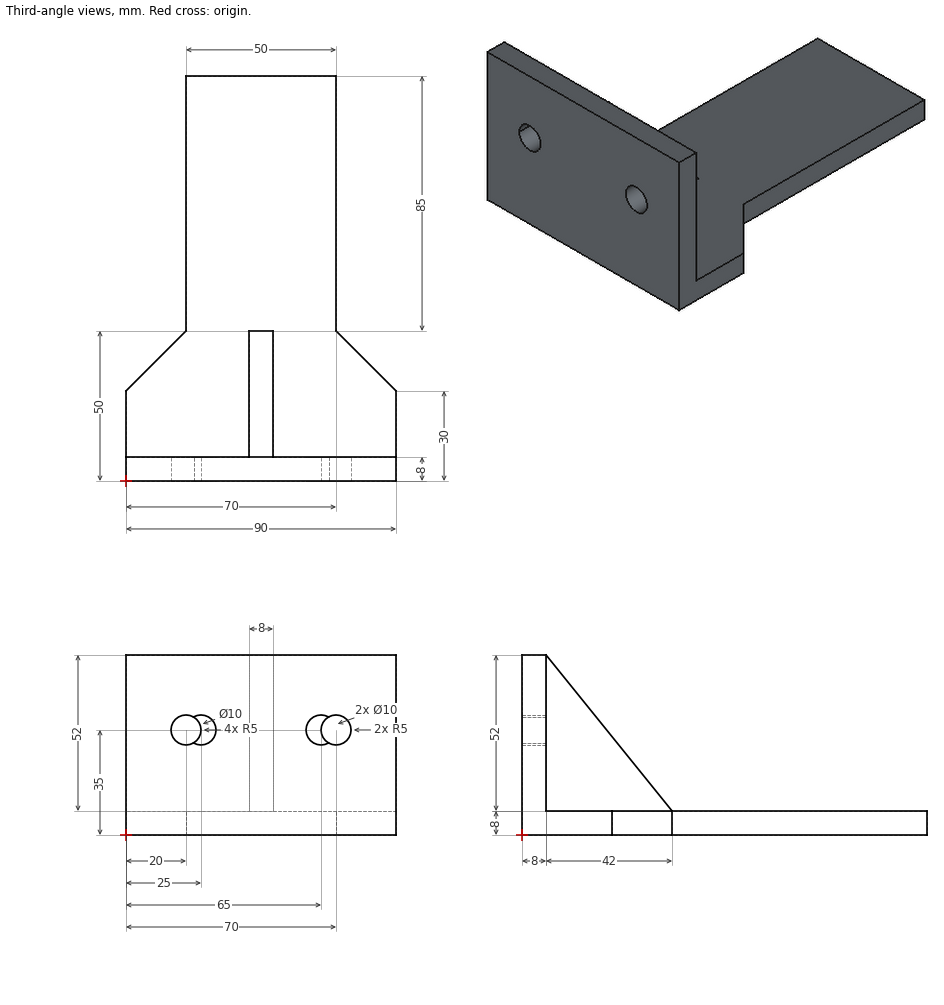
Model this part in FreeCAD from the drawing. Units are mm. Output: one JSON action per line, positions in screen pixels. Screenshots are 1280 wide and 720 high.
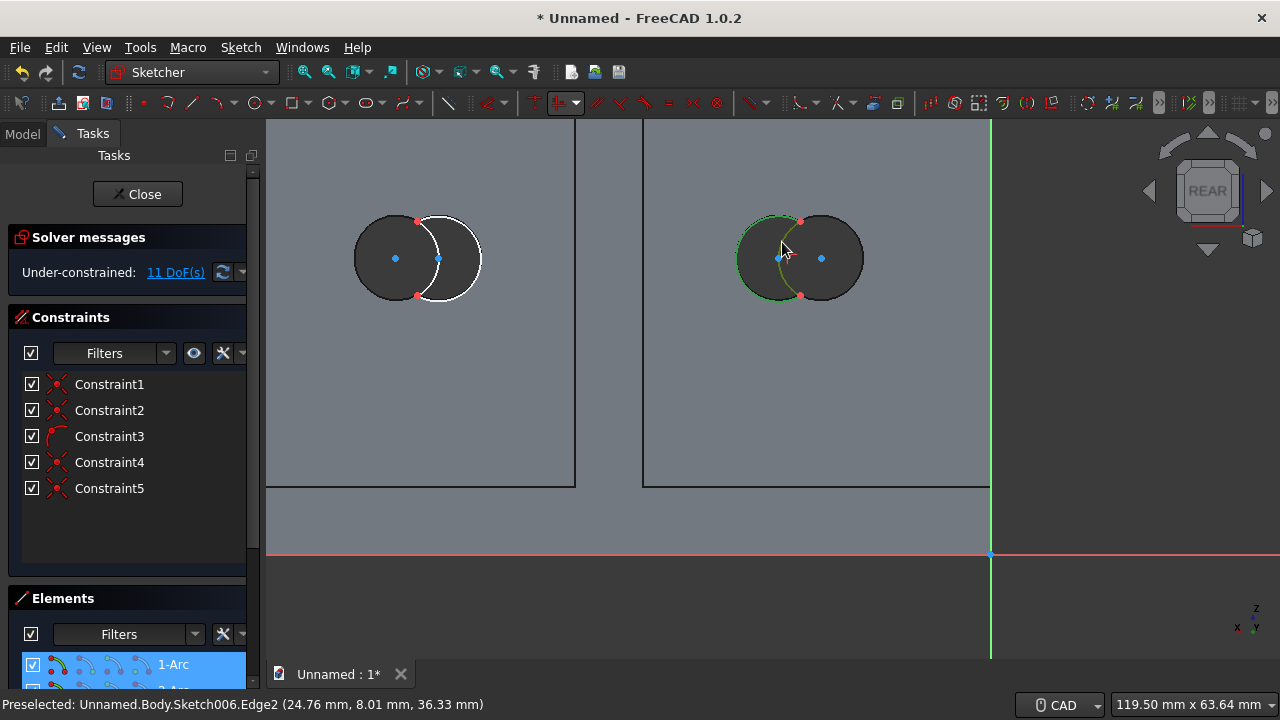
{"action": "left_click", "coordinate": [435, 276]}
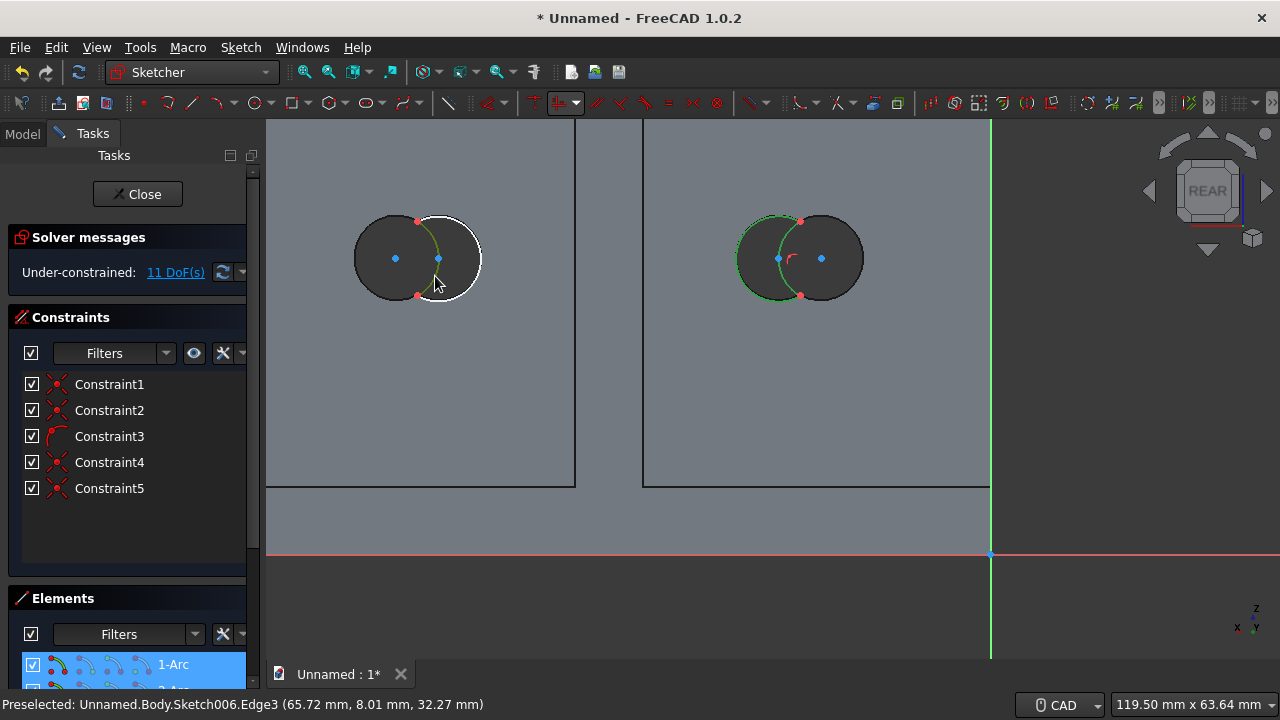
{"action": "left_click", "coordinate": [467, 290]}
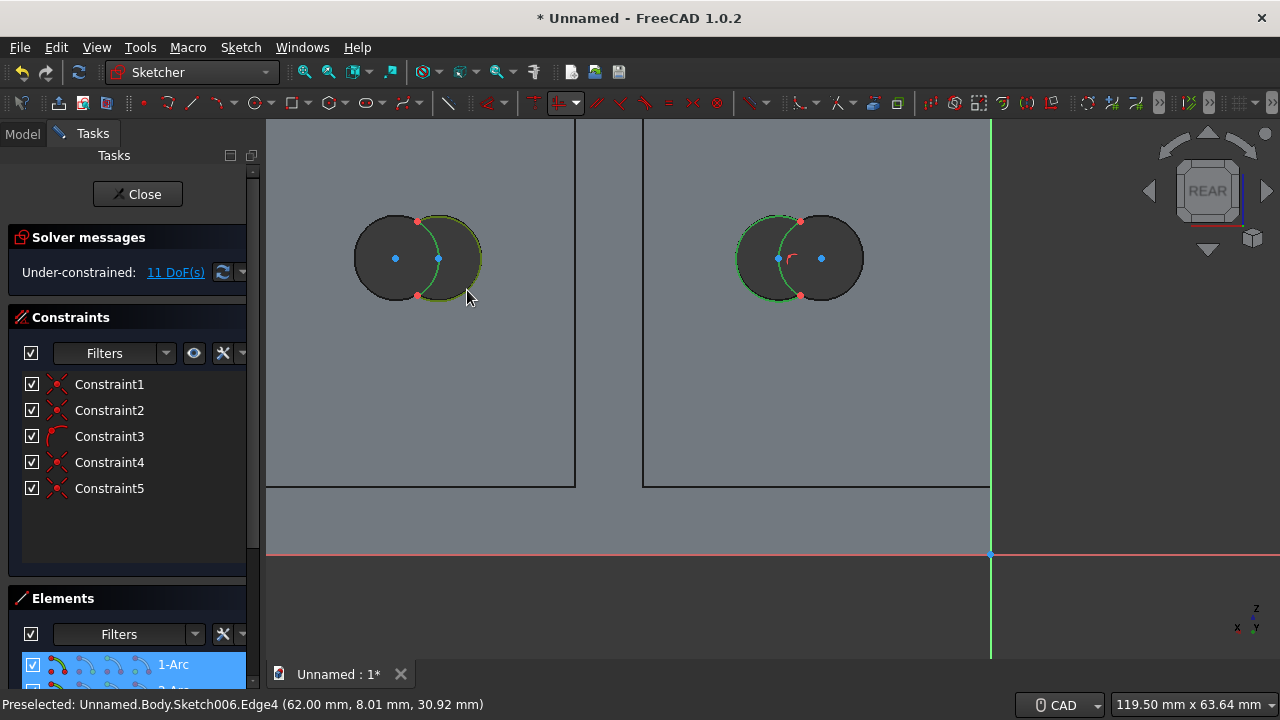
{"action": "left_click", "coordinate": [670, 104]}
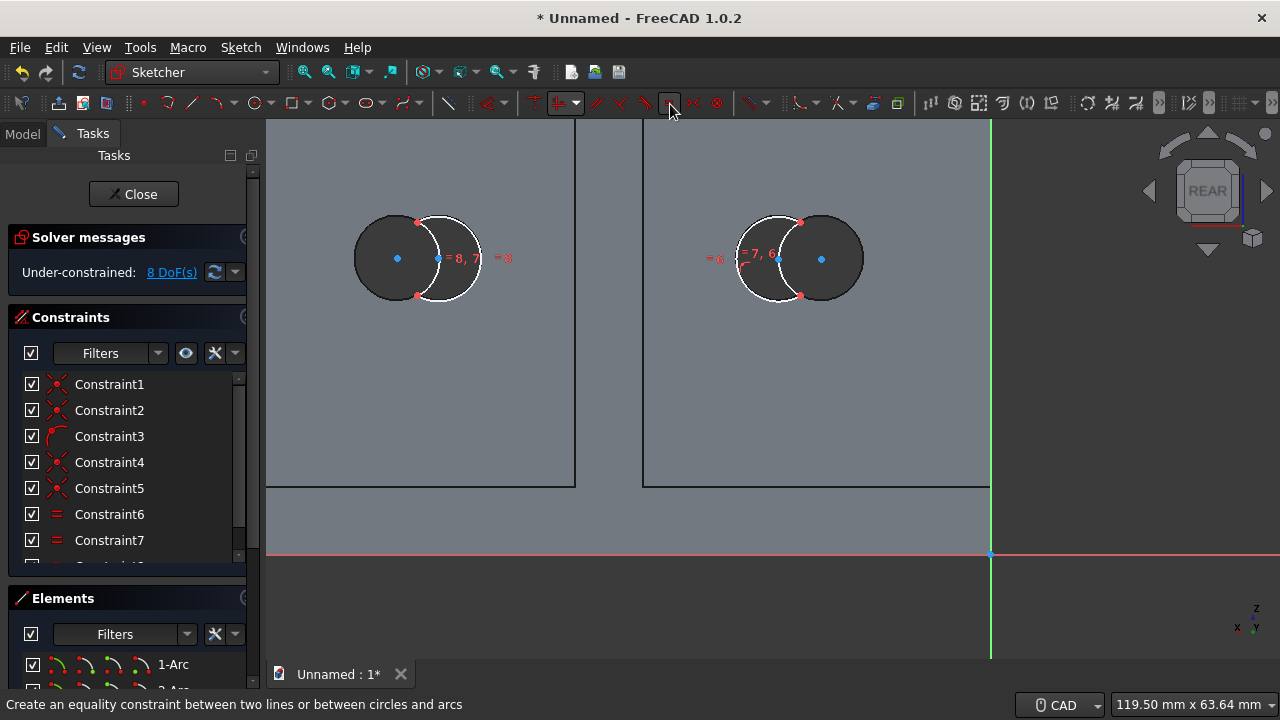
{"action": "left_click", "coordinate": [488, 104]}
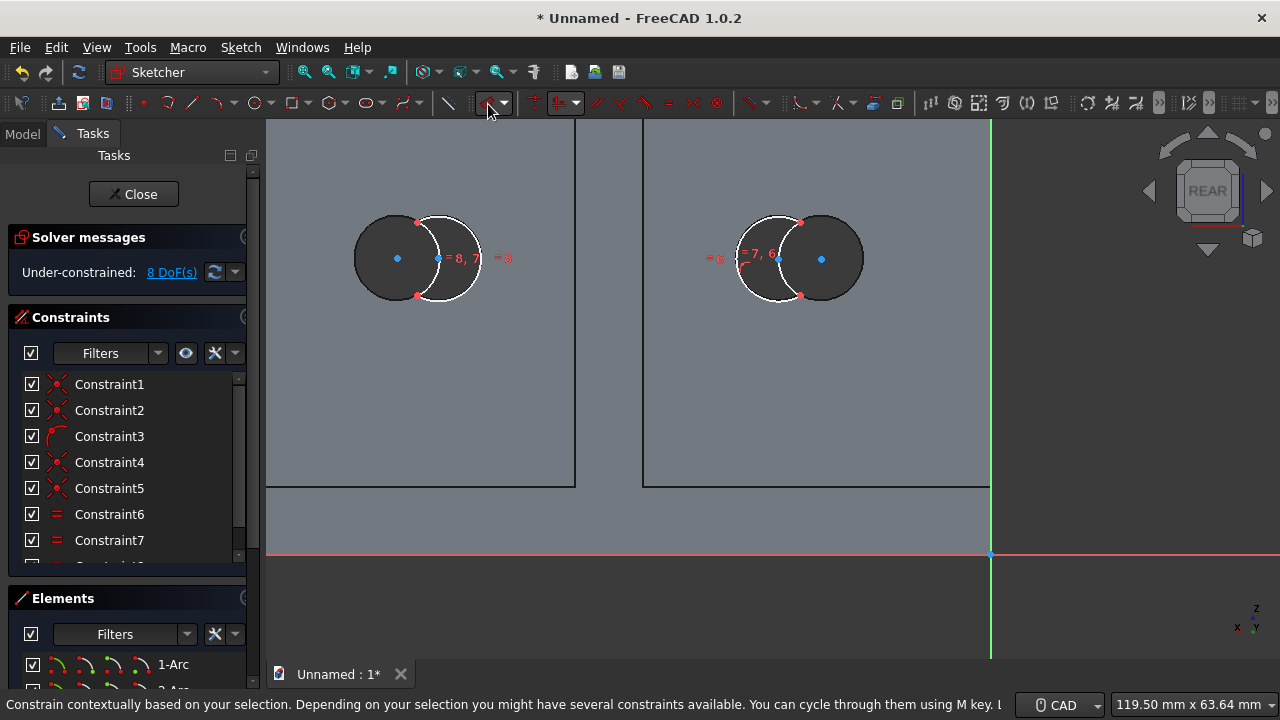
{"action": "left_click", "coordinate": [750, 228]}
{"action": "left_click", "coordinate": [728, 204]}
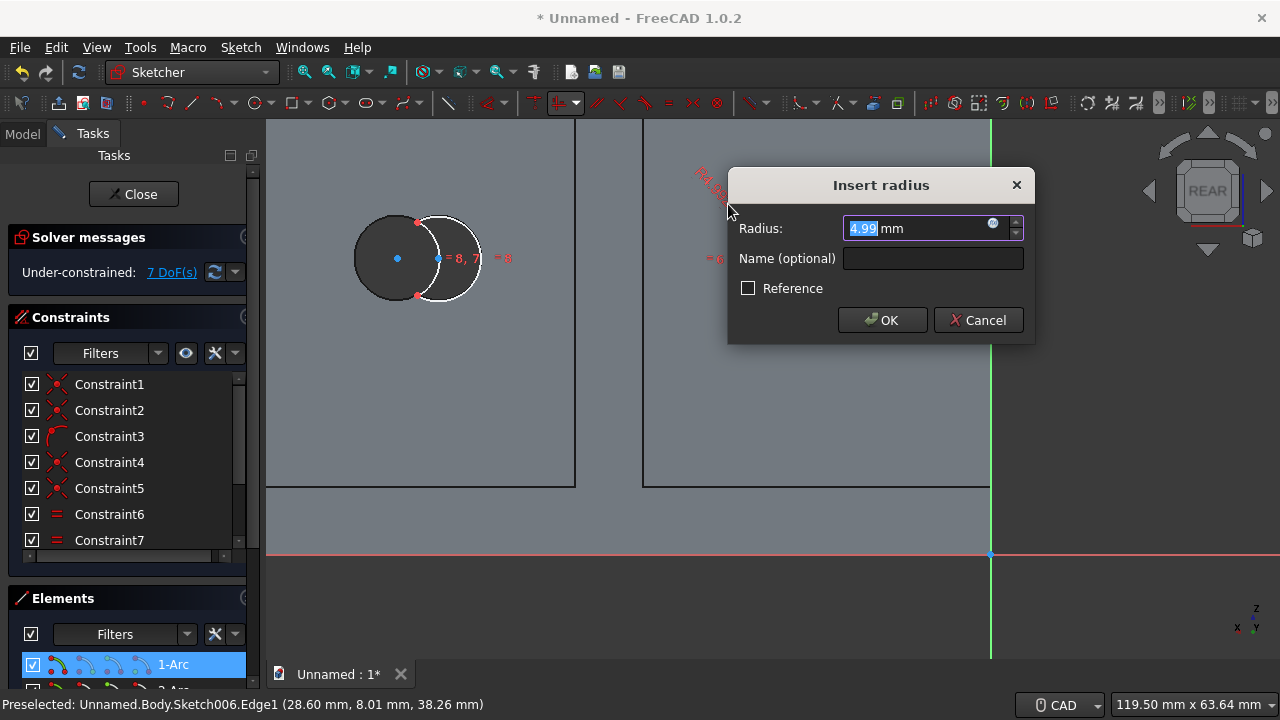
{"action": "type", "text": "5"}
{"action": "key", "text": "Return"}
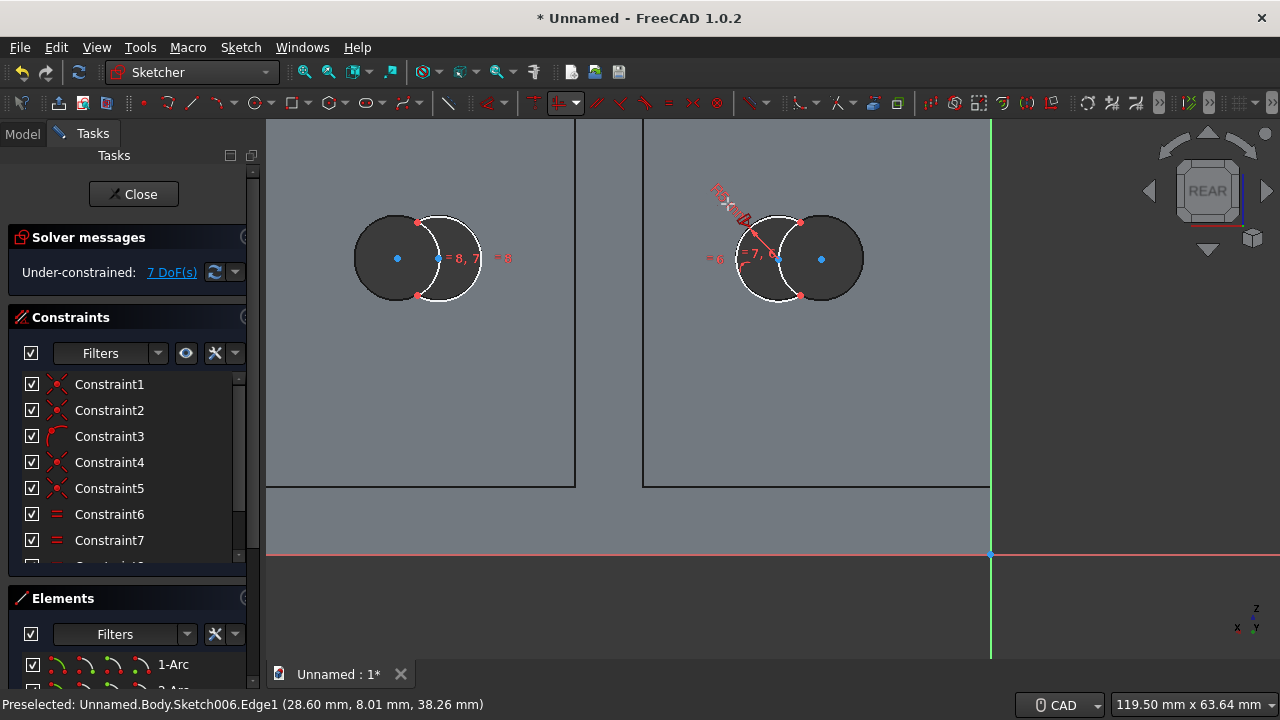
{"action": "left_click", "coordinate": [779, 259]}
{"action": "left_click", "coordinate": [885, 589]}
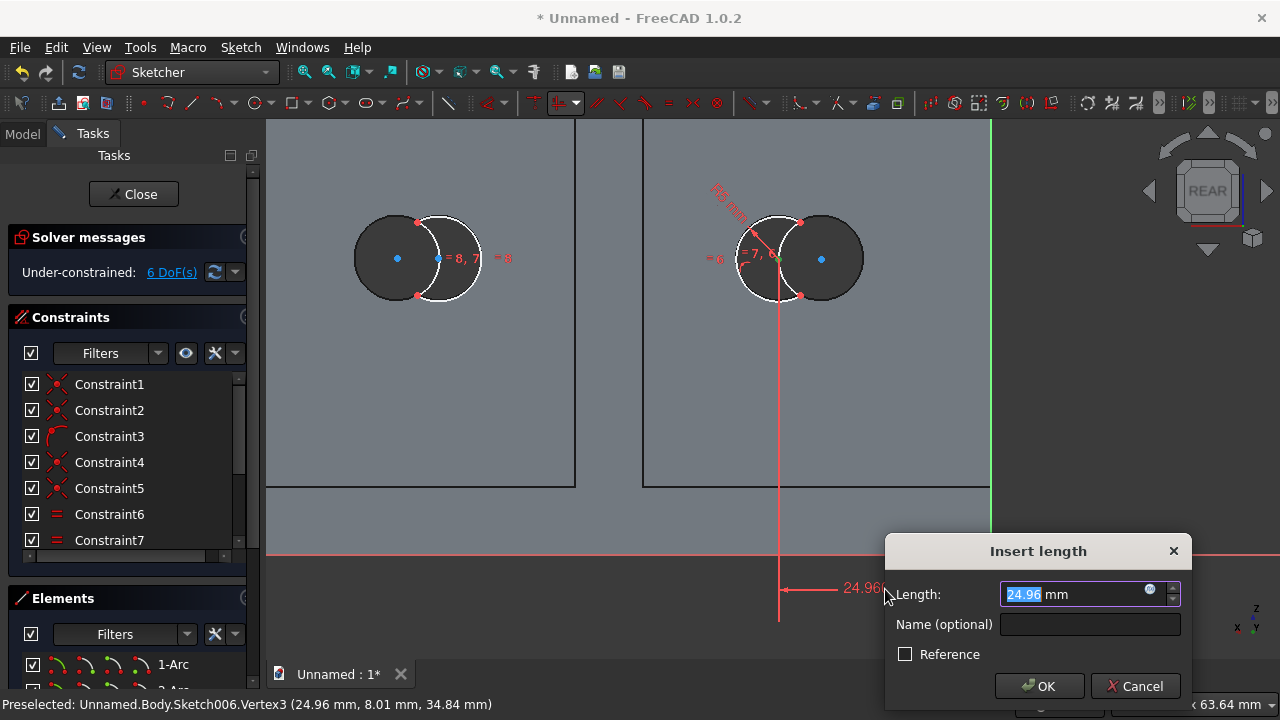
{"action": "type", "text": "25"}
{"action": "key", "text": "Return"}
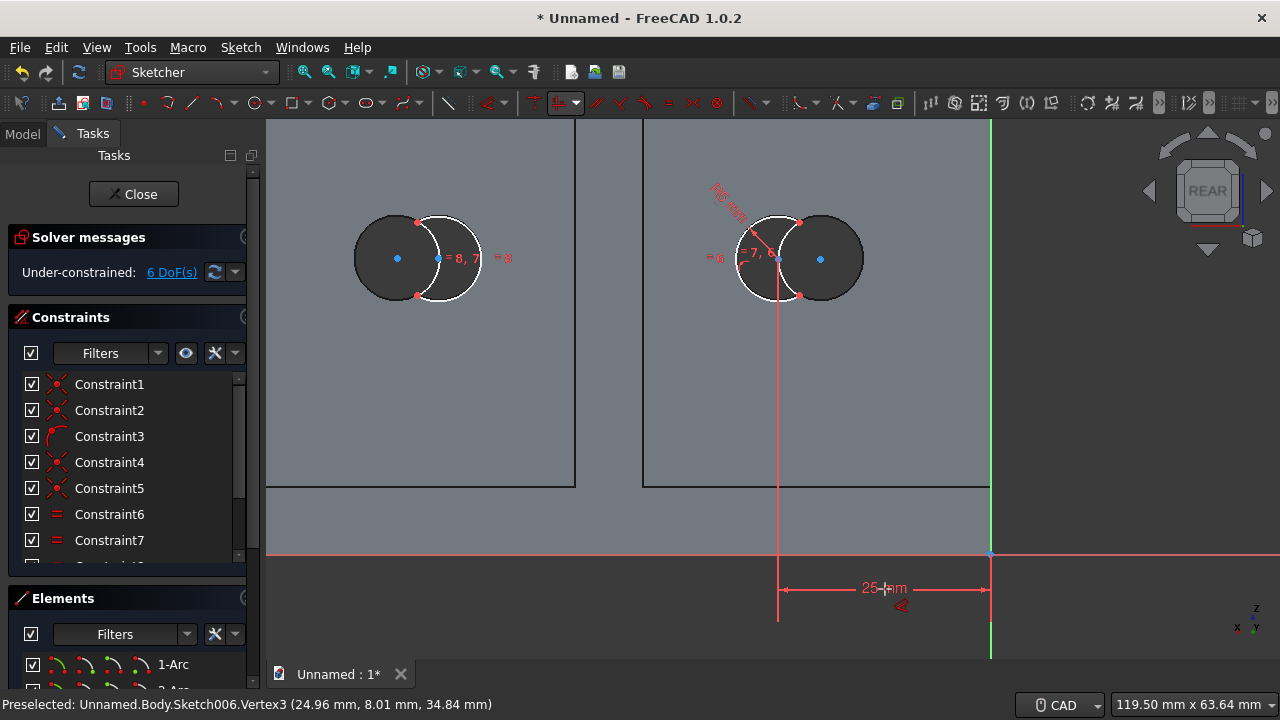
{"action": "left_click", "coordinate": [778, 259]}
{"action": "left_click", "coordinate": [1025, 407]}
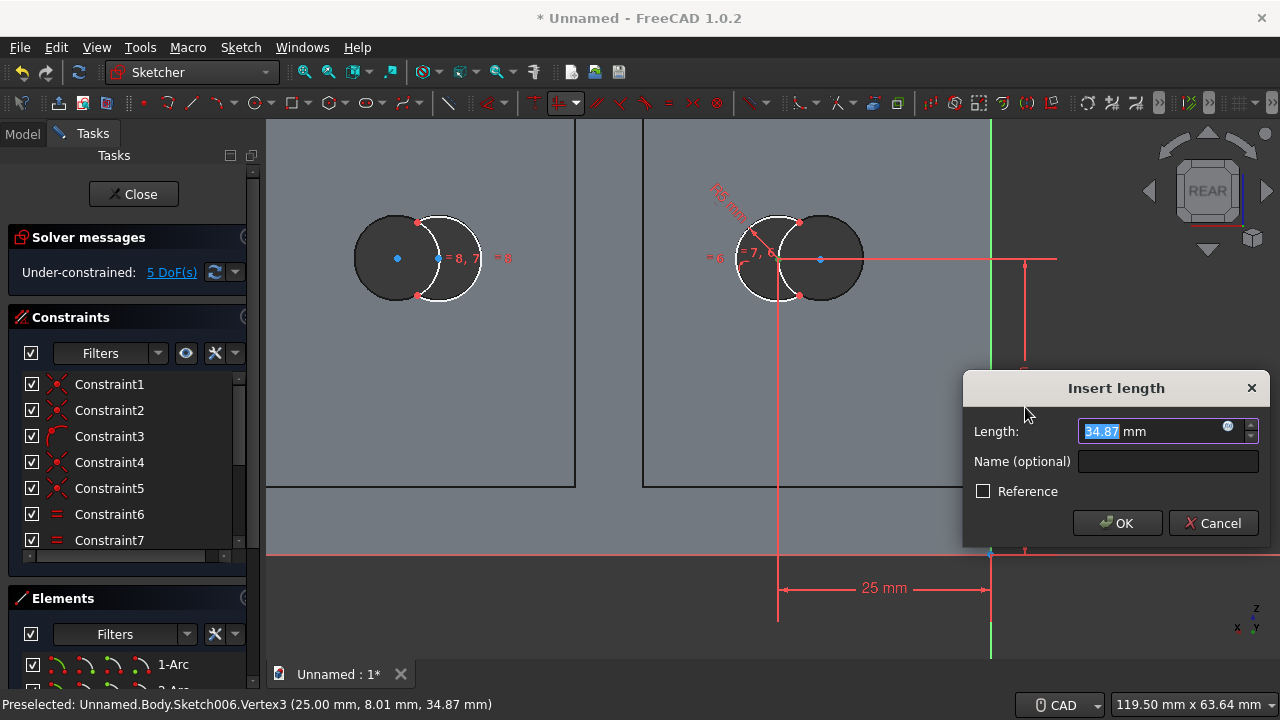
{"action": "type", "text": "35"}
{"action": "key", "text": "Return"}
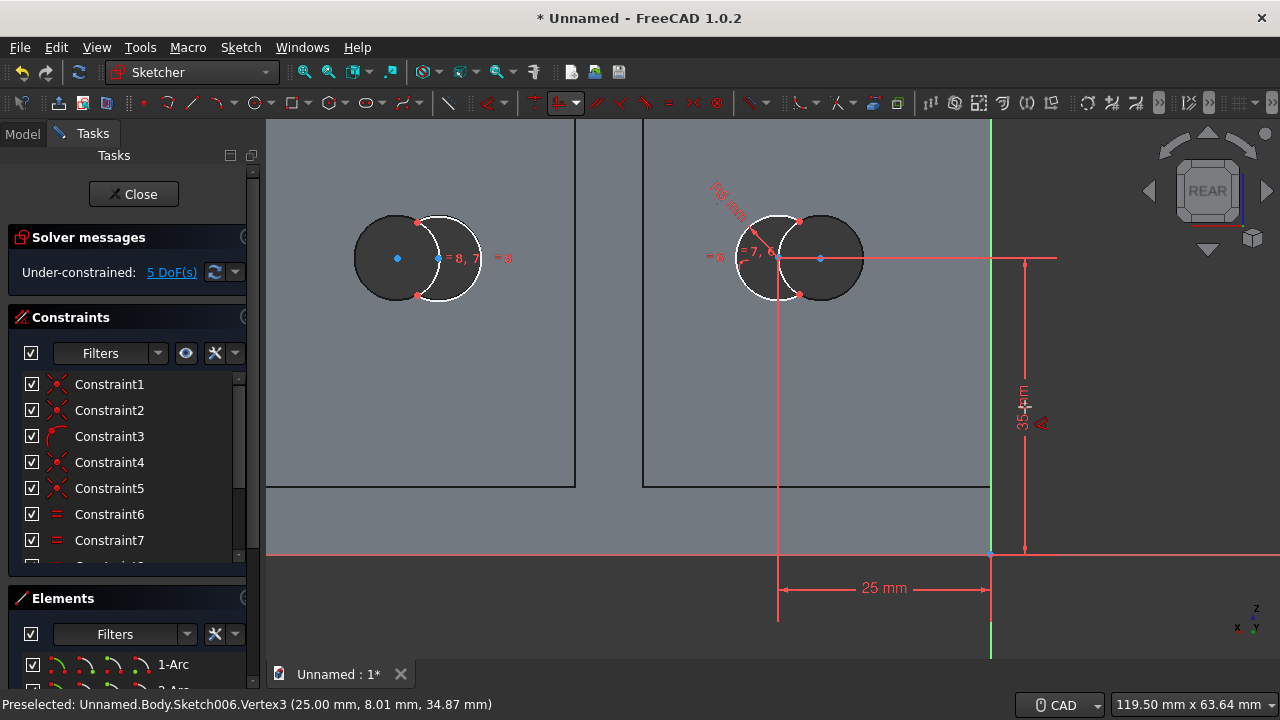
{"action": "left_click", "coordinate": [821, 258]}
{"action": "left_click", "coordinate": [1025, 338]}